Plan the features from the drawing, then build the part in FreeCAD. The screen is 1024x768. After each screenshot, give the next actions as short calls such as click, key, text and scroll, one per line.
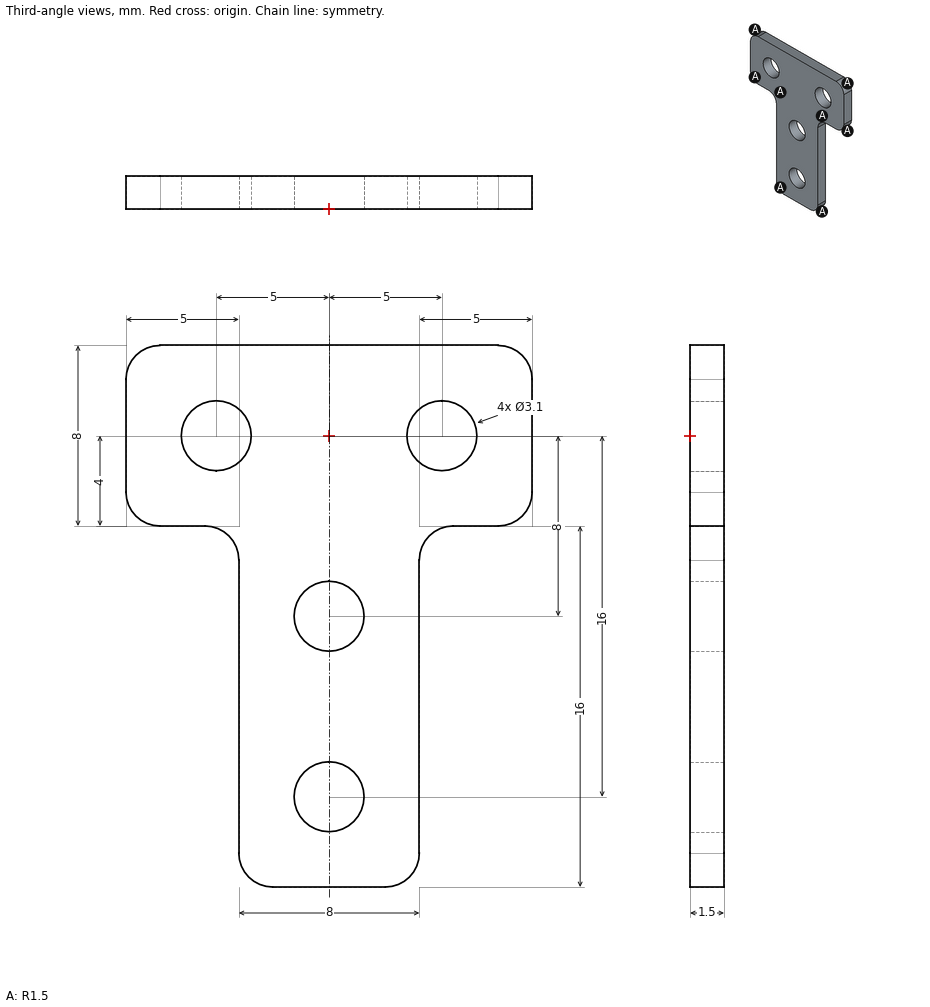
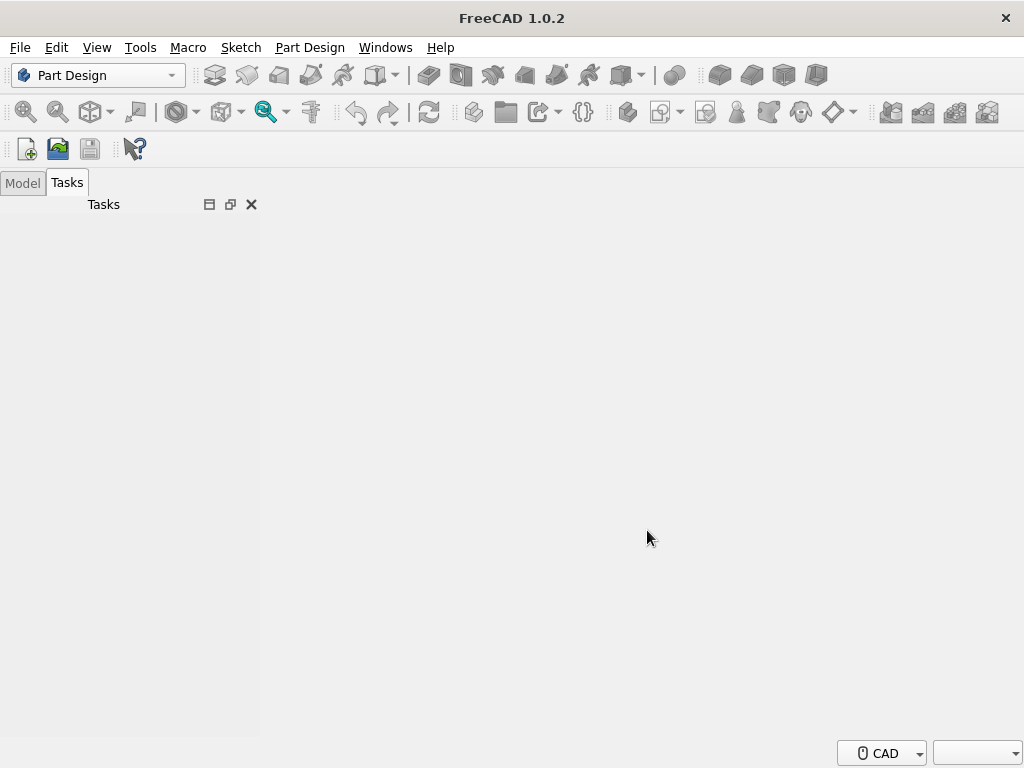
click(26, 150)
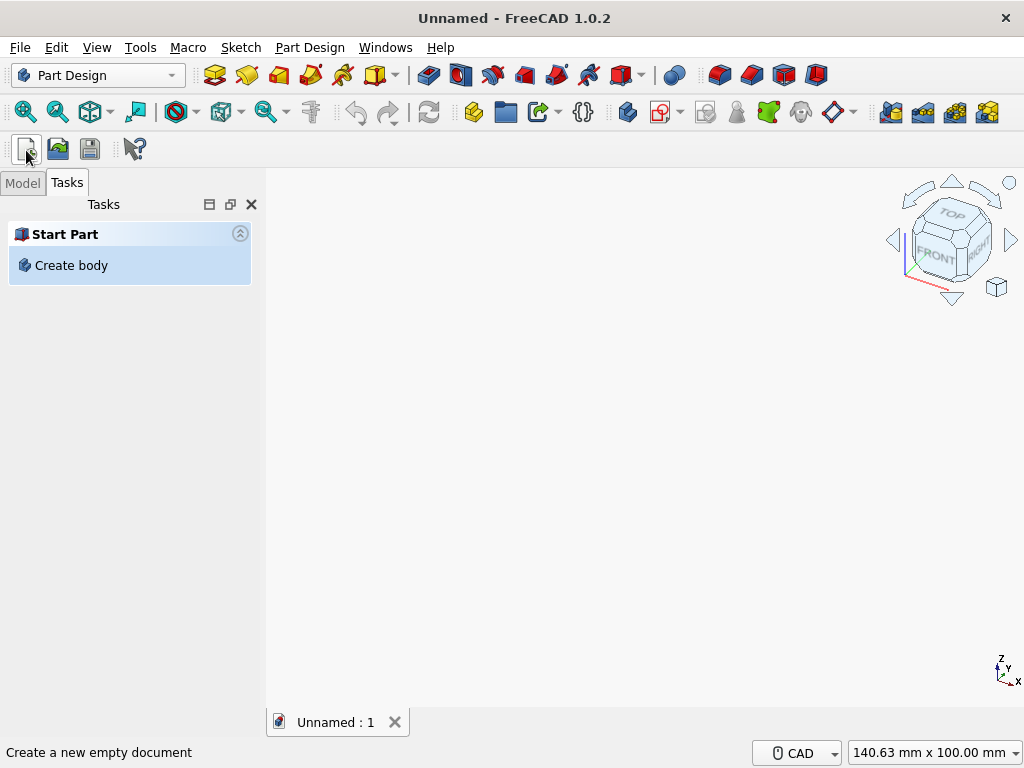
click(660, 112)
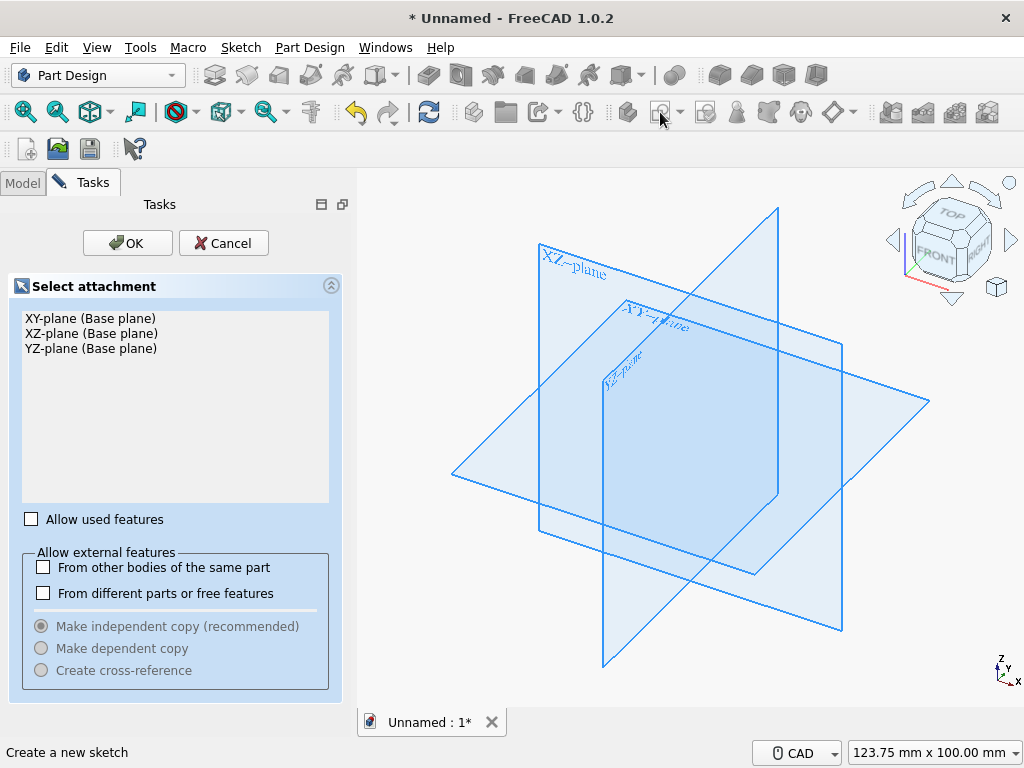
click(82, 334)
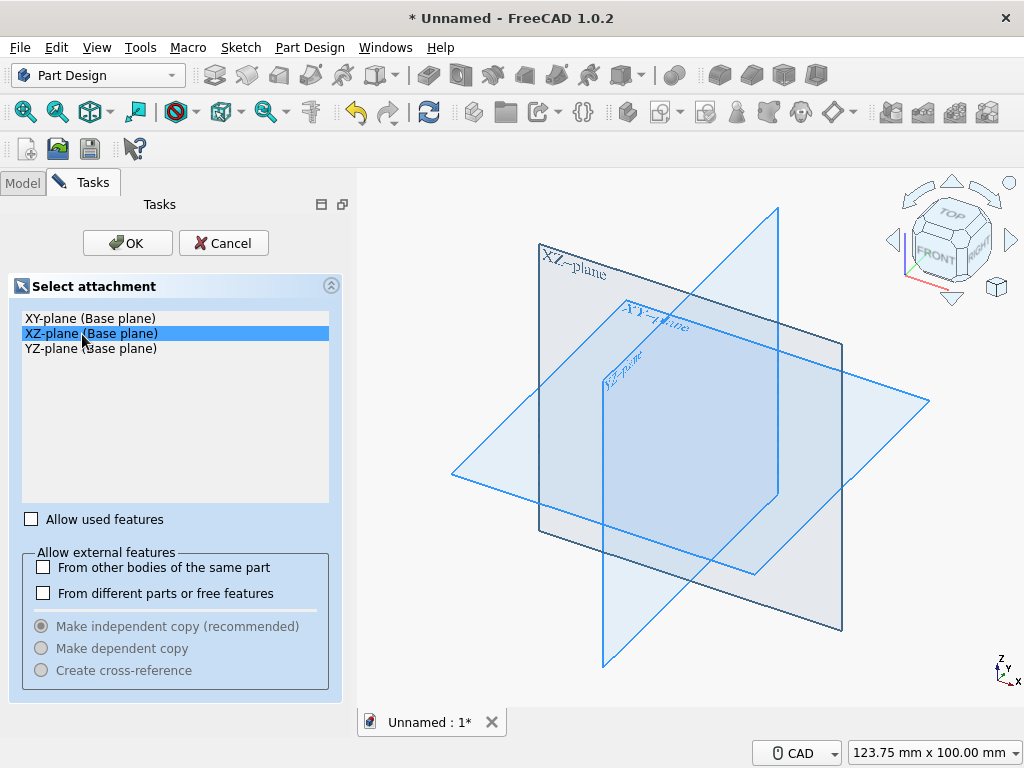
click(128, 243)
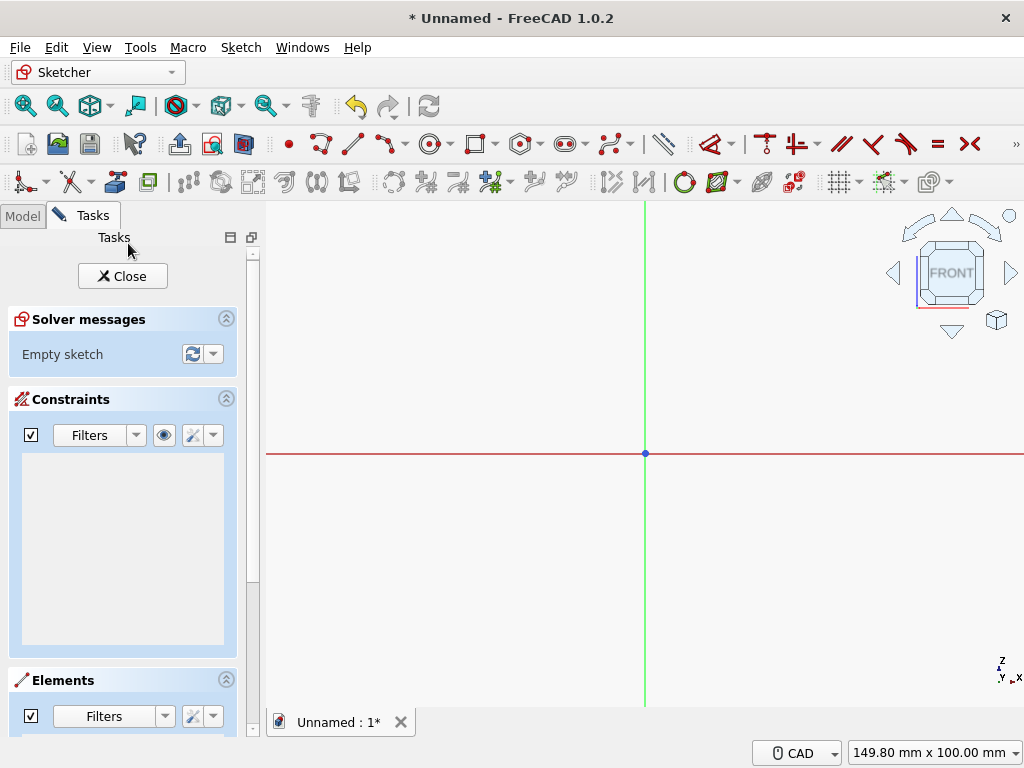
scroll(685, 518, up, 5)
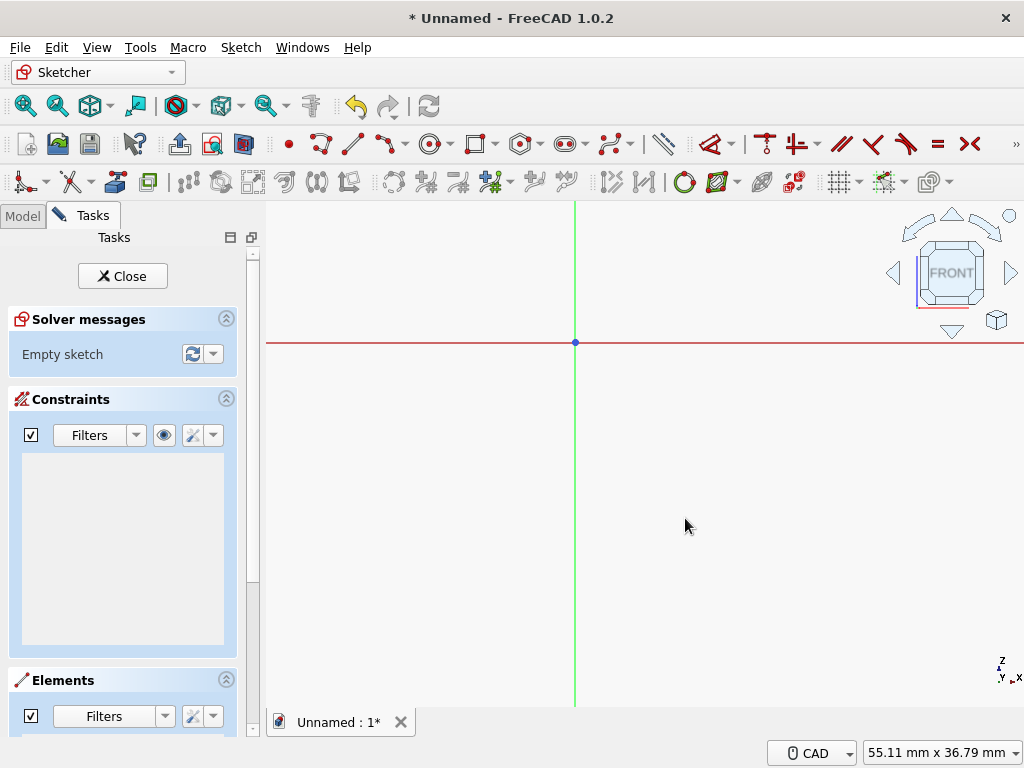
click(322, 144)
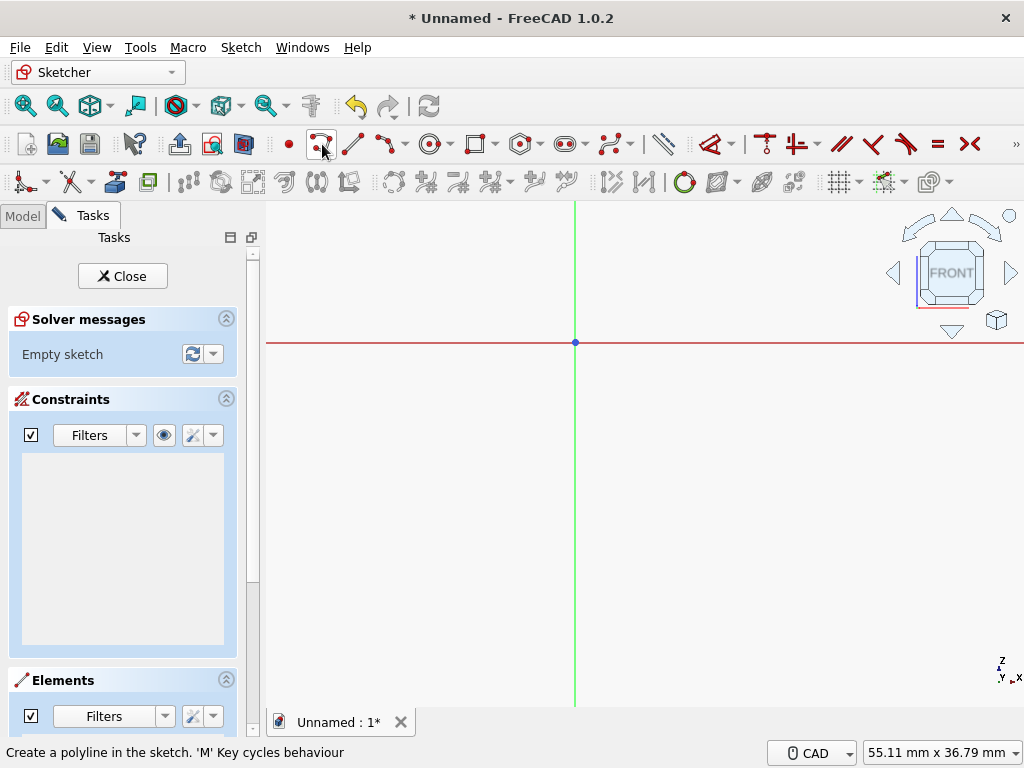
click(520, 398)
click(452, 398)
click(452, 288)
click(699, 288)
click(699, 398)
click(630, 398)
click(630, 618)
click(520, 618)
click(520, 399)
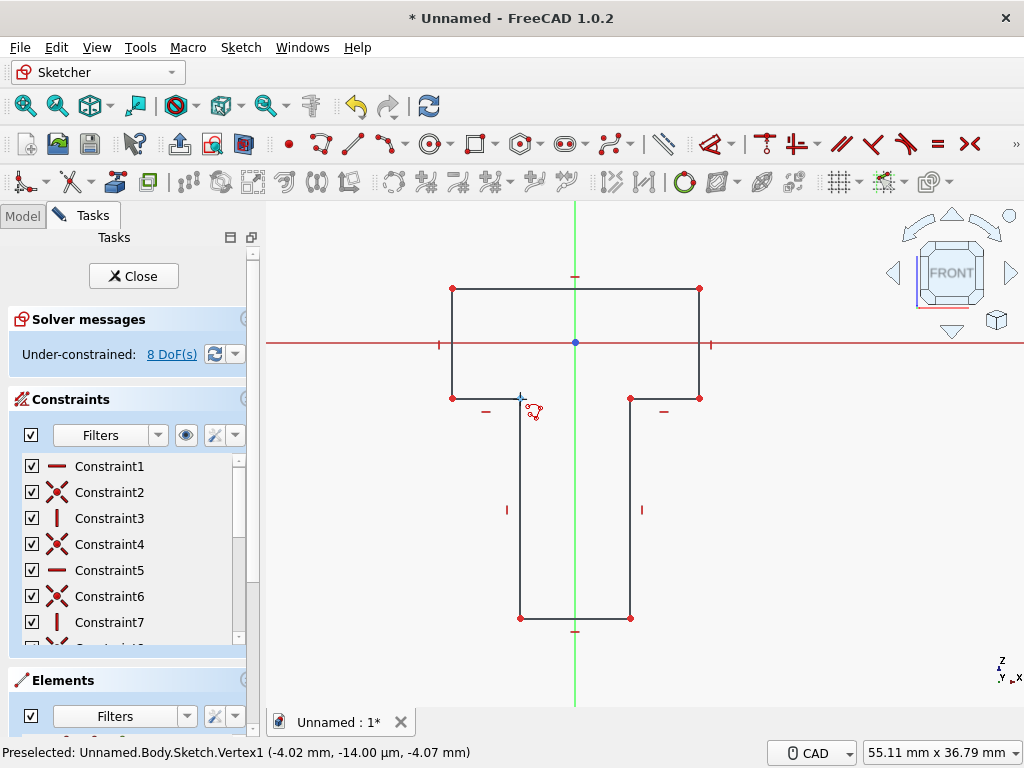
click(430, 144)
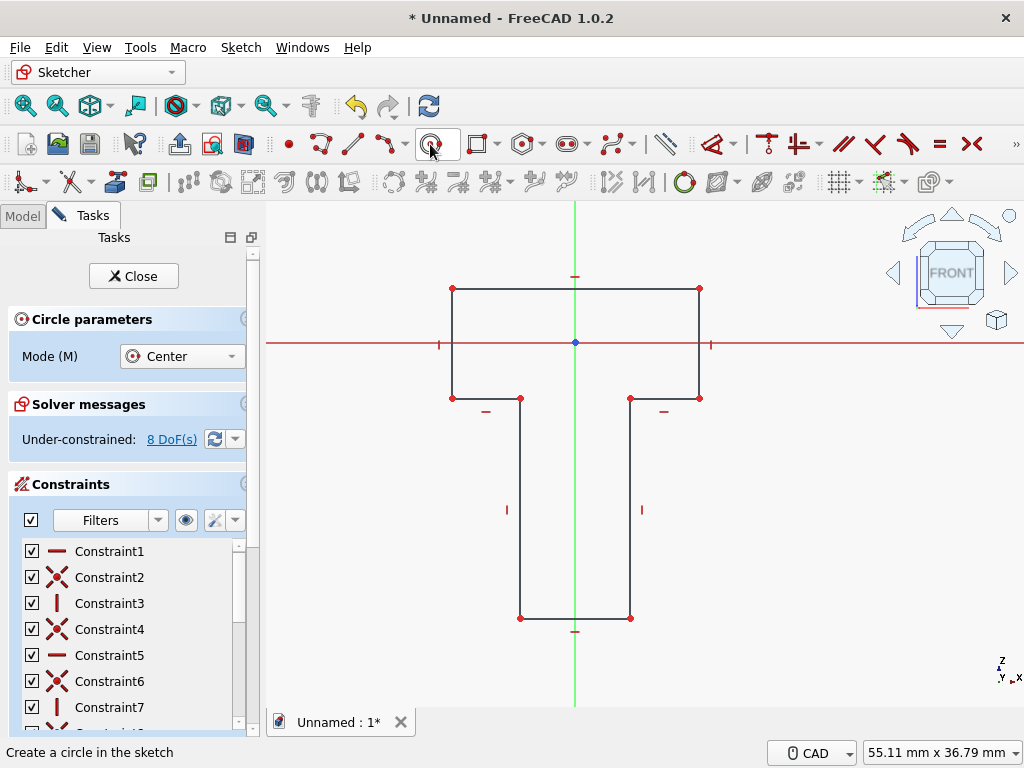
click(644, 343)
click(659, 328)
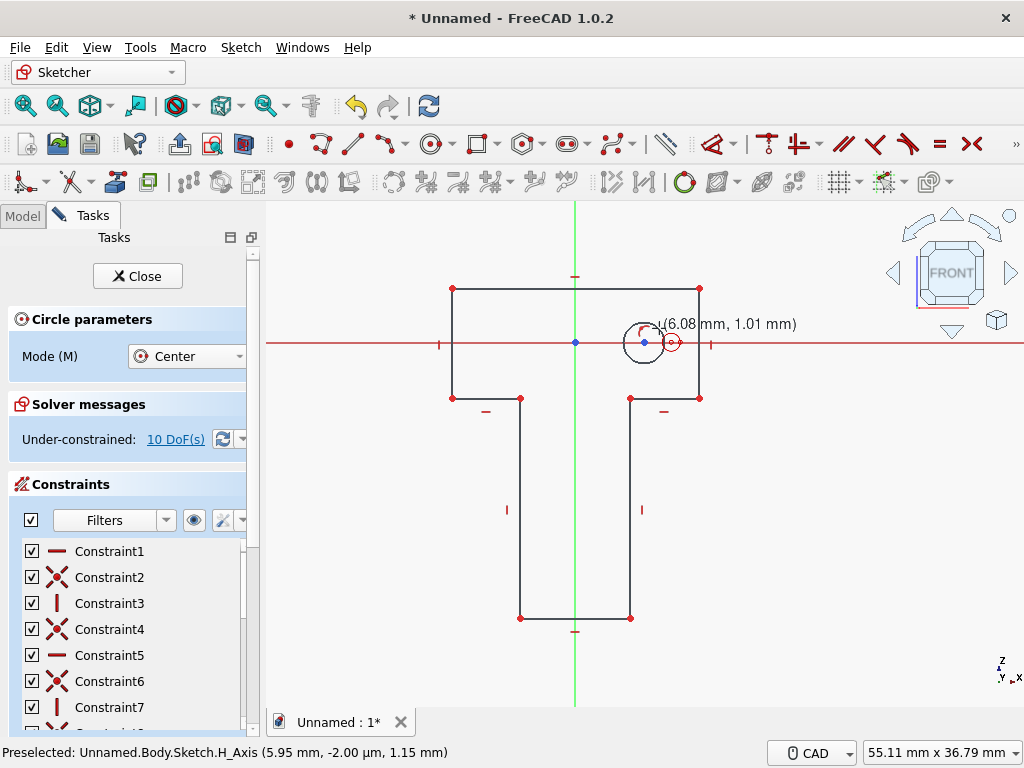
click(507, 343)
click(522, 328)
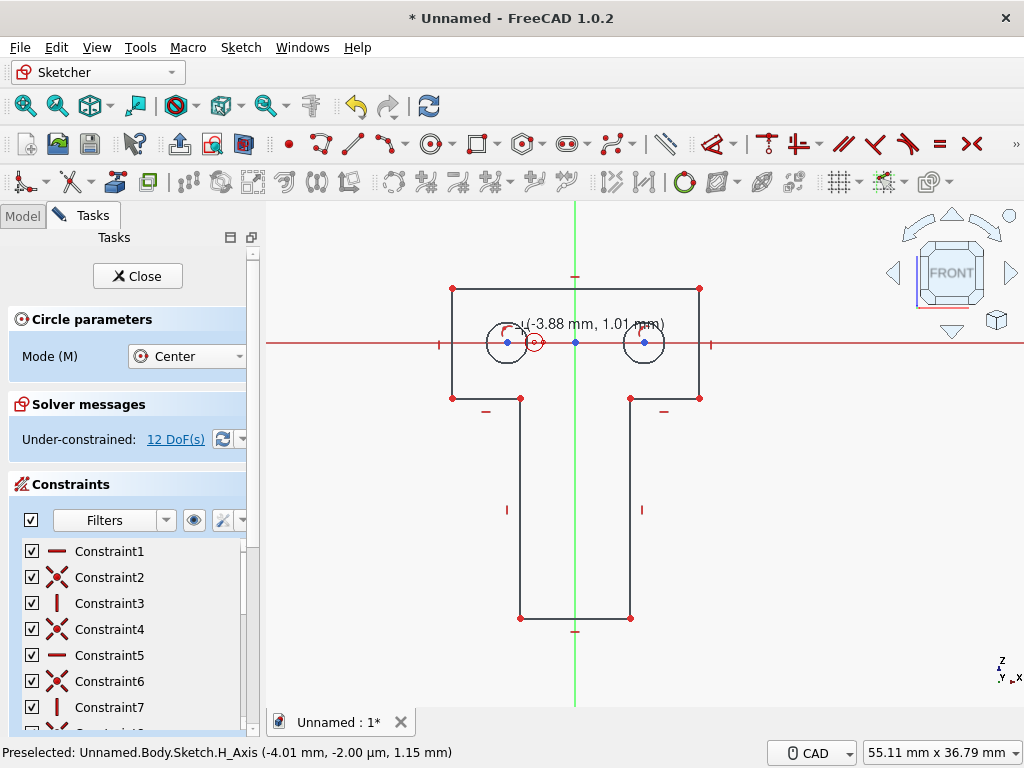
click(575, 453)
click(590, 438)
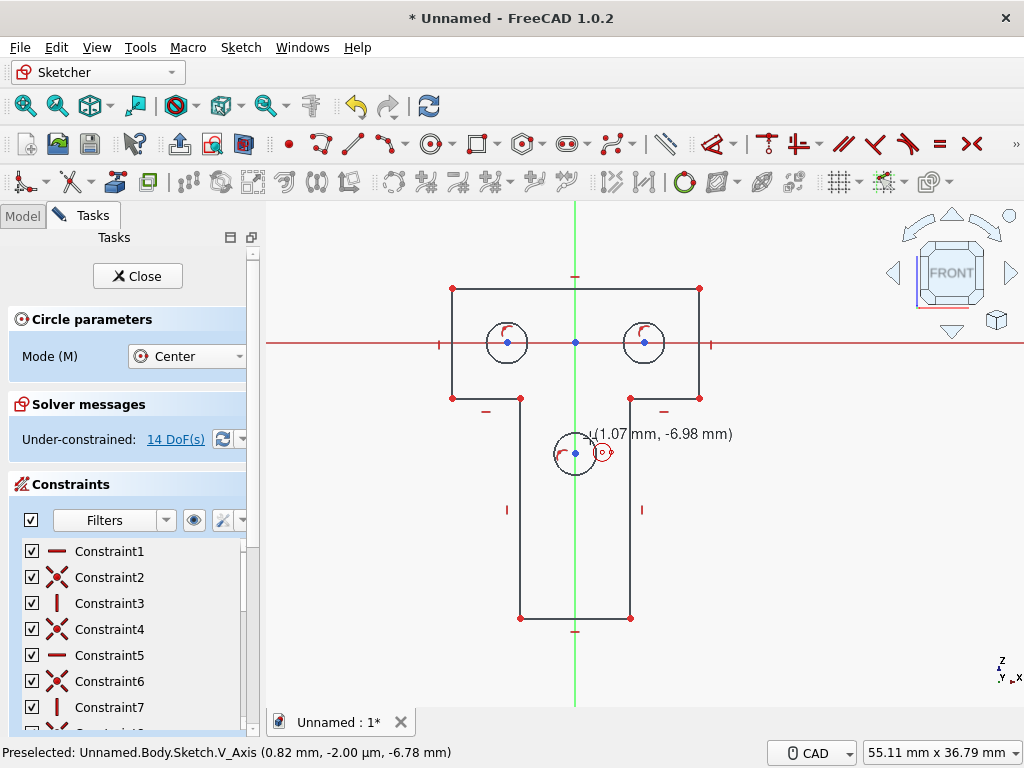
click(575, 563)
click(590, 548)
key(Escape)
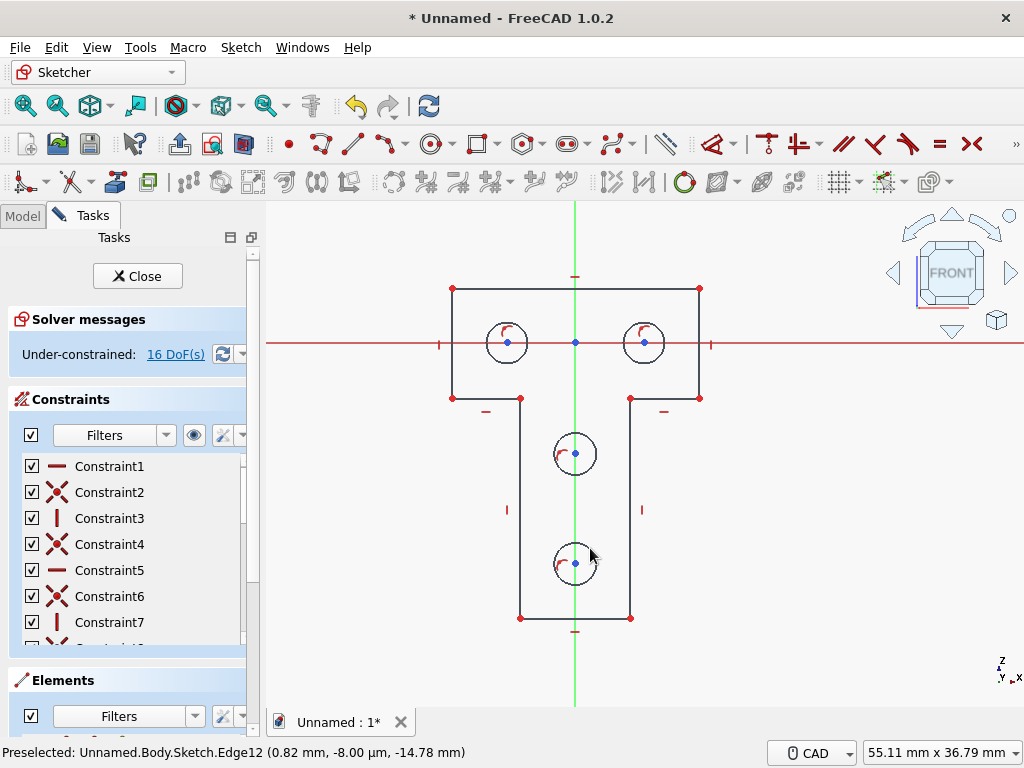
click(658, 328)